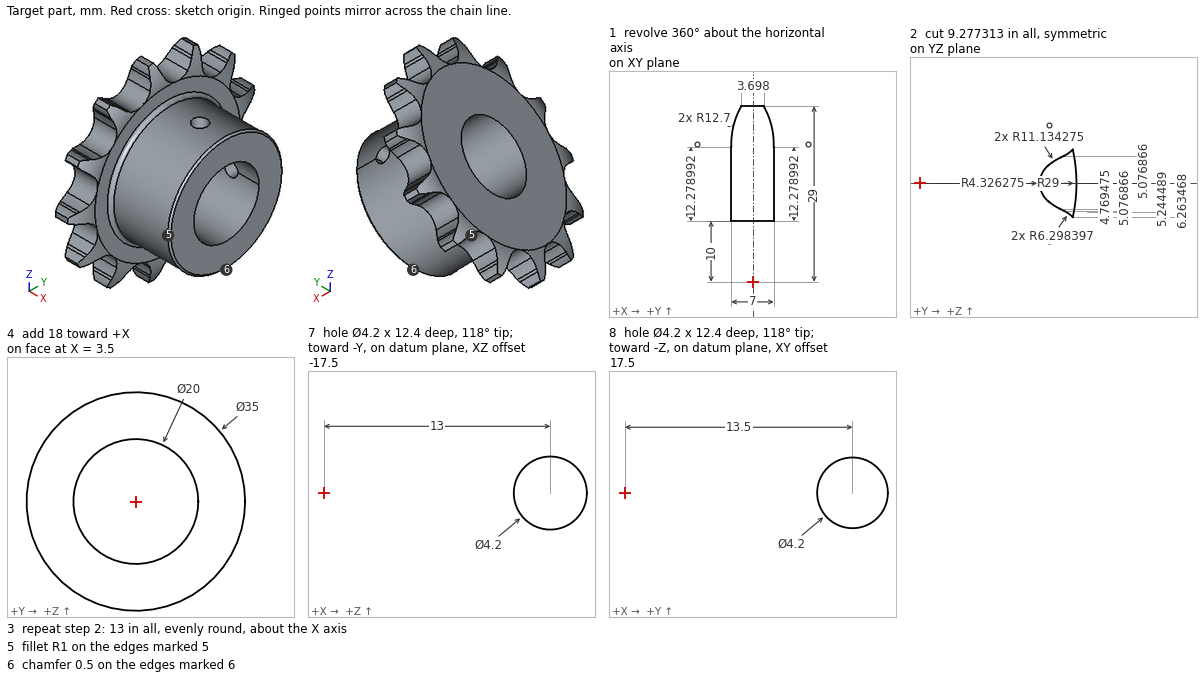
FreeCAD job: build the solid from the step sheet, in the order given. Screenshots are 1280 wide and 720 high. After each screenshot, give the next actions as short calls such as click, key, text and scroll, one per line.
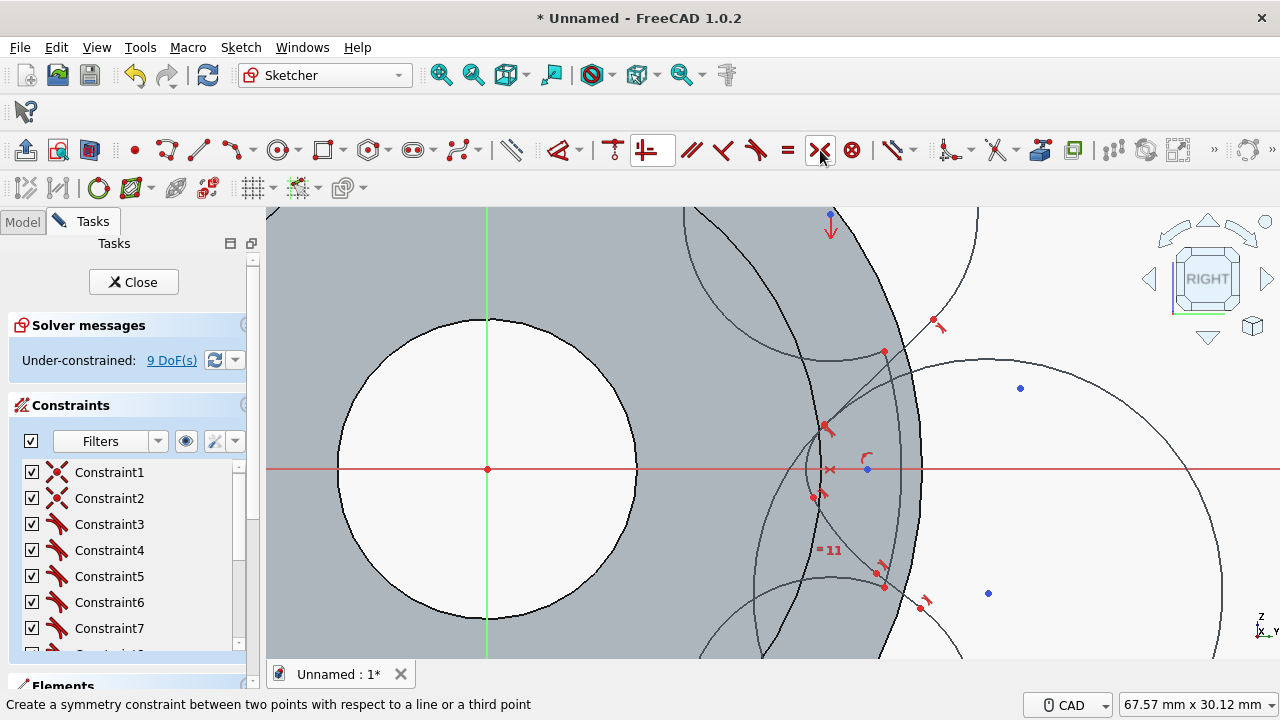
click(558, 150)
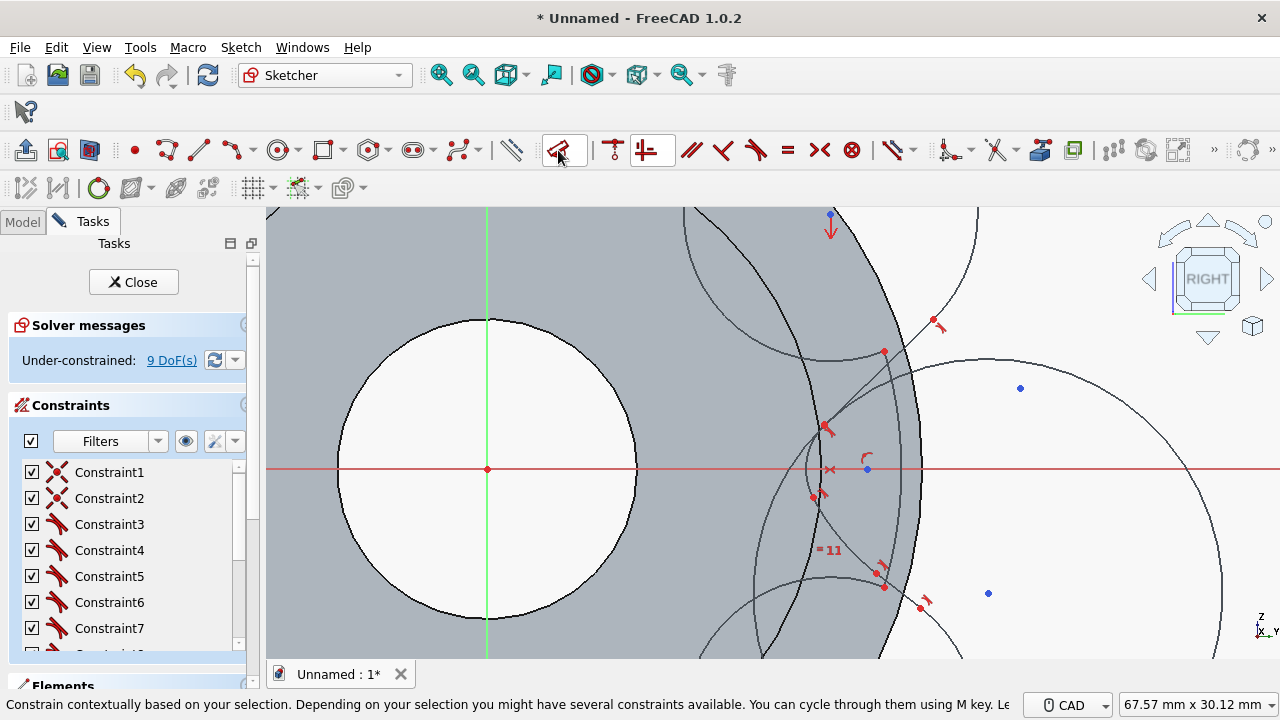
click(723, 625)
click(699, 603)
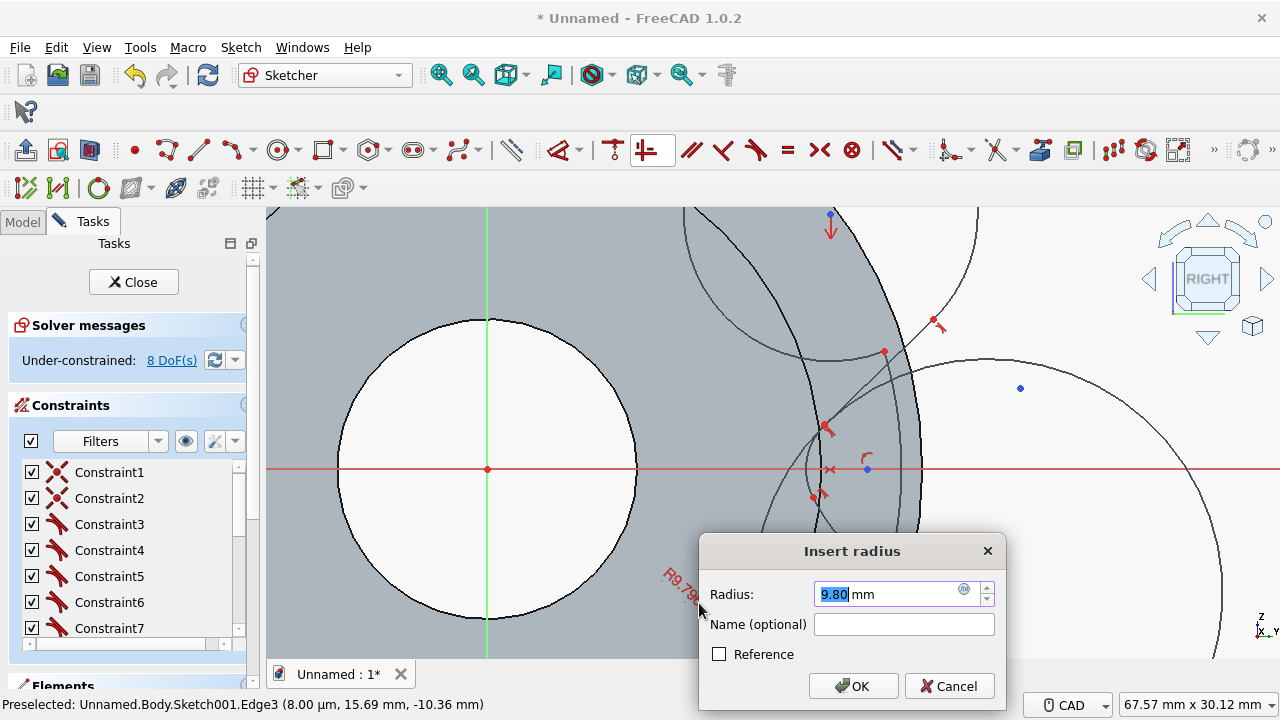
text(6.298397)
key(Return)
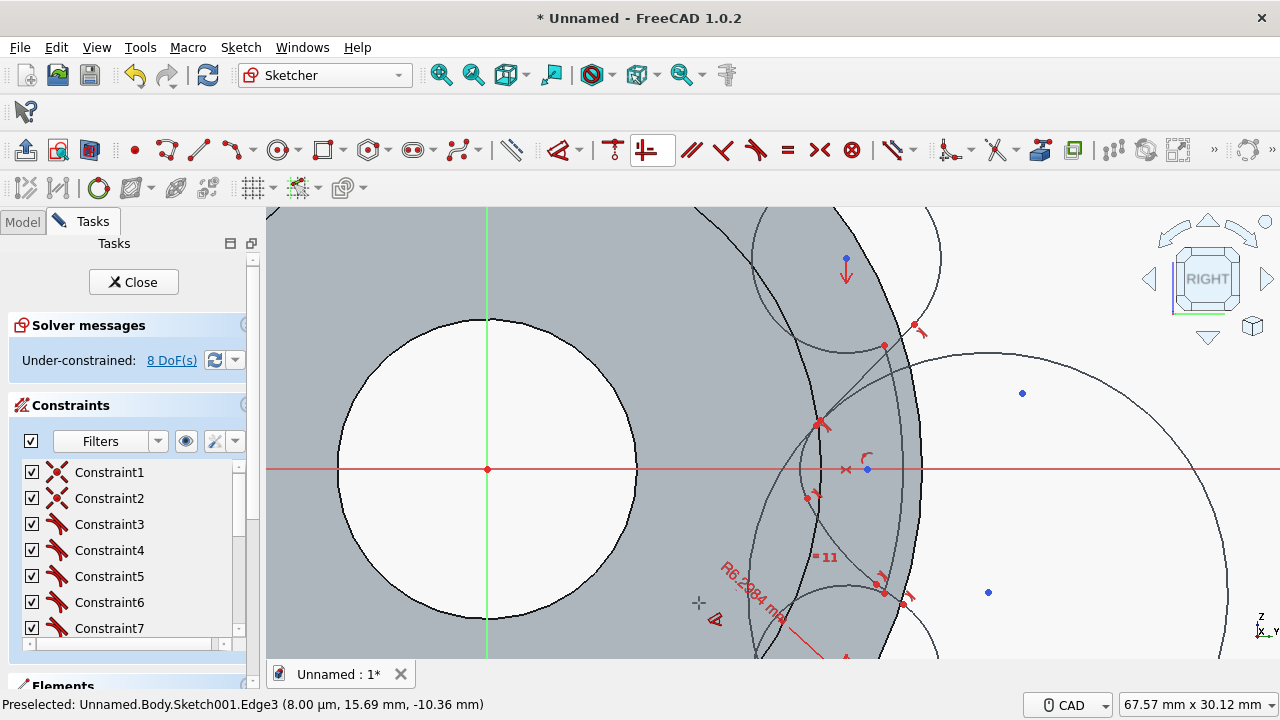
click(900, 519)
click(932, 523)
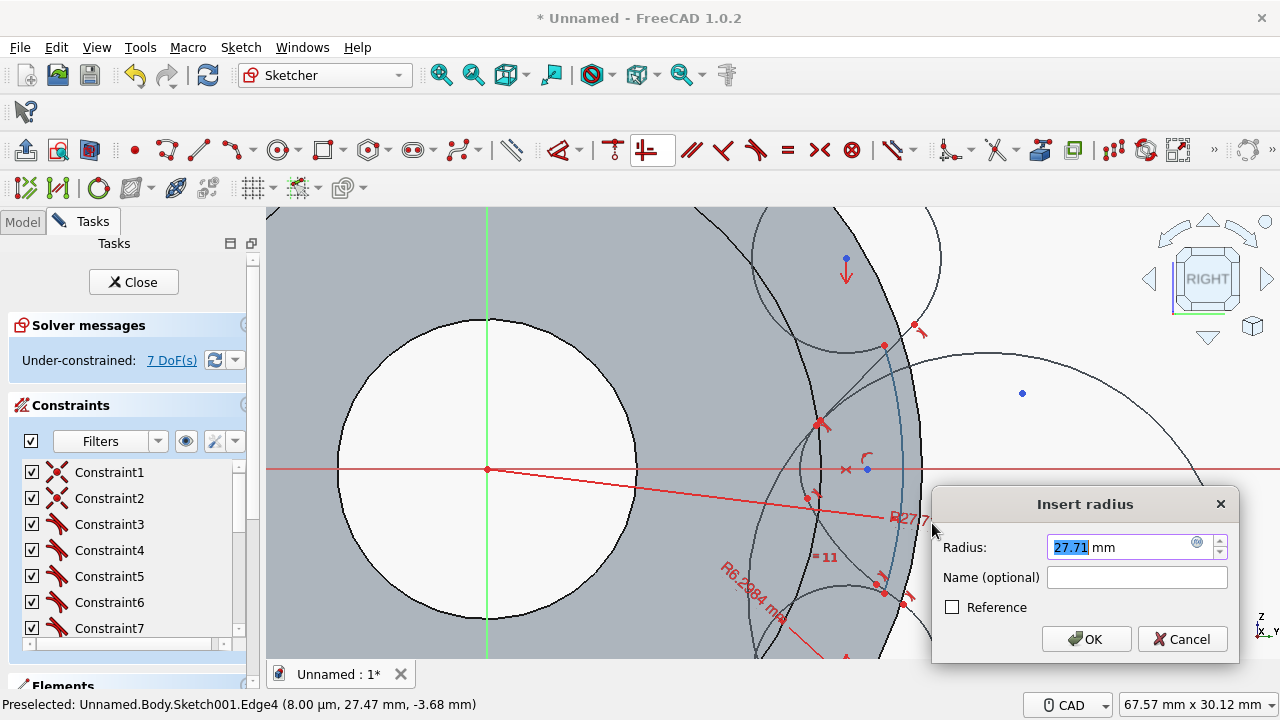
text(29)
key(Return)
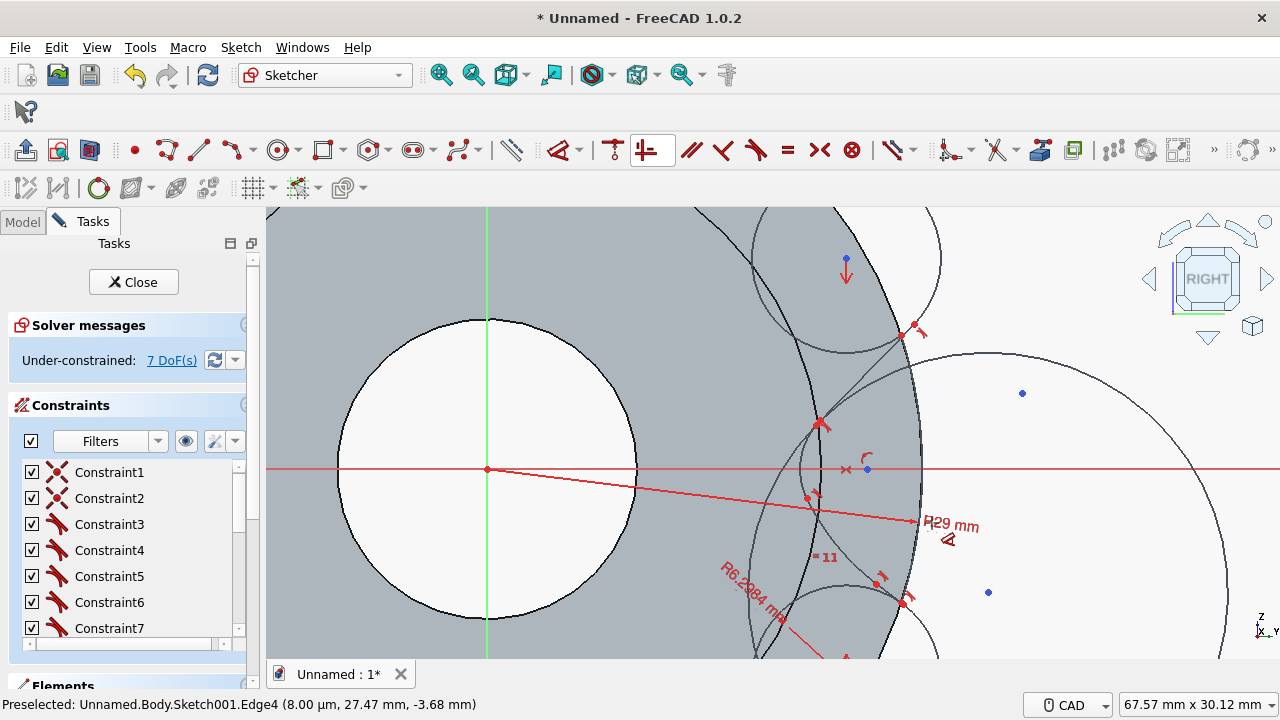
click(1099, 380)
click(1114, 352)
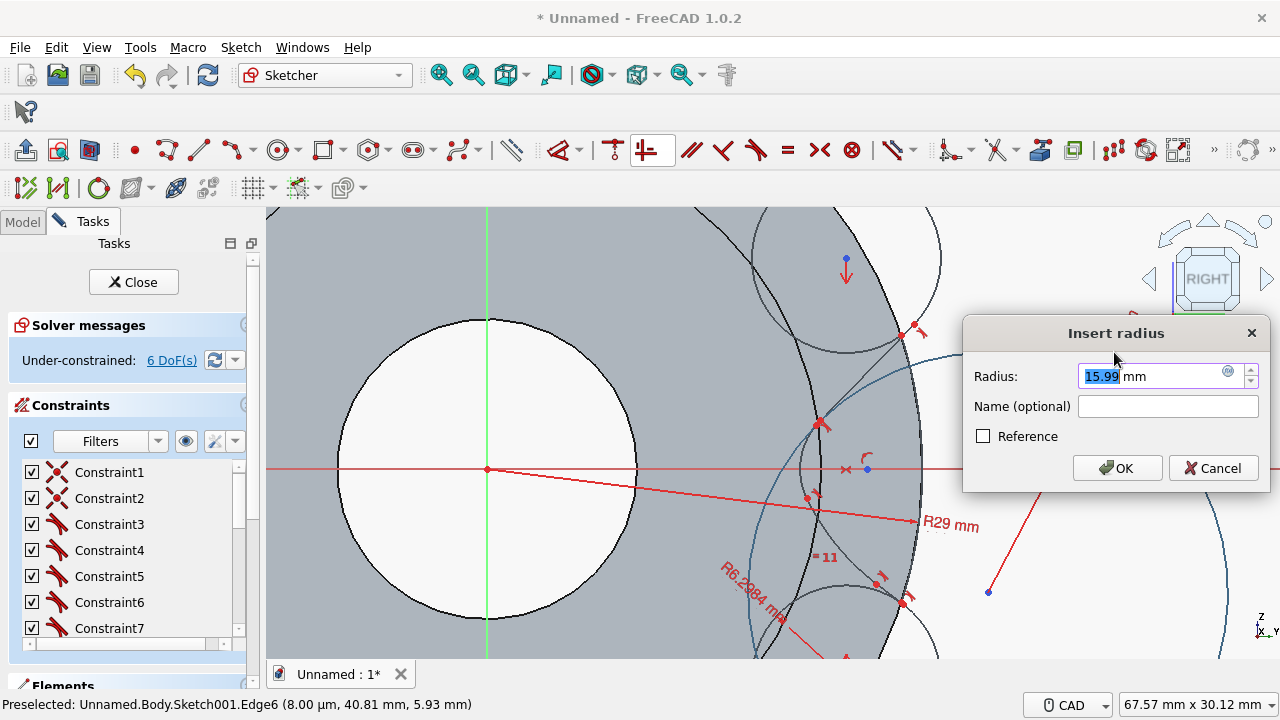
text(11.134275)
key(Return)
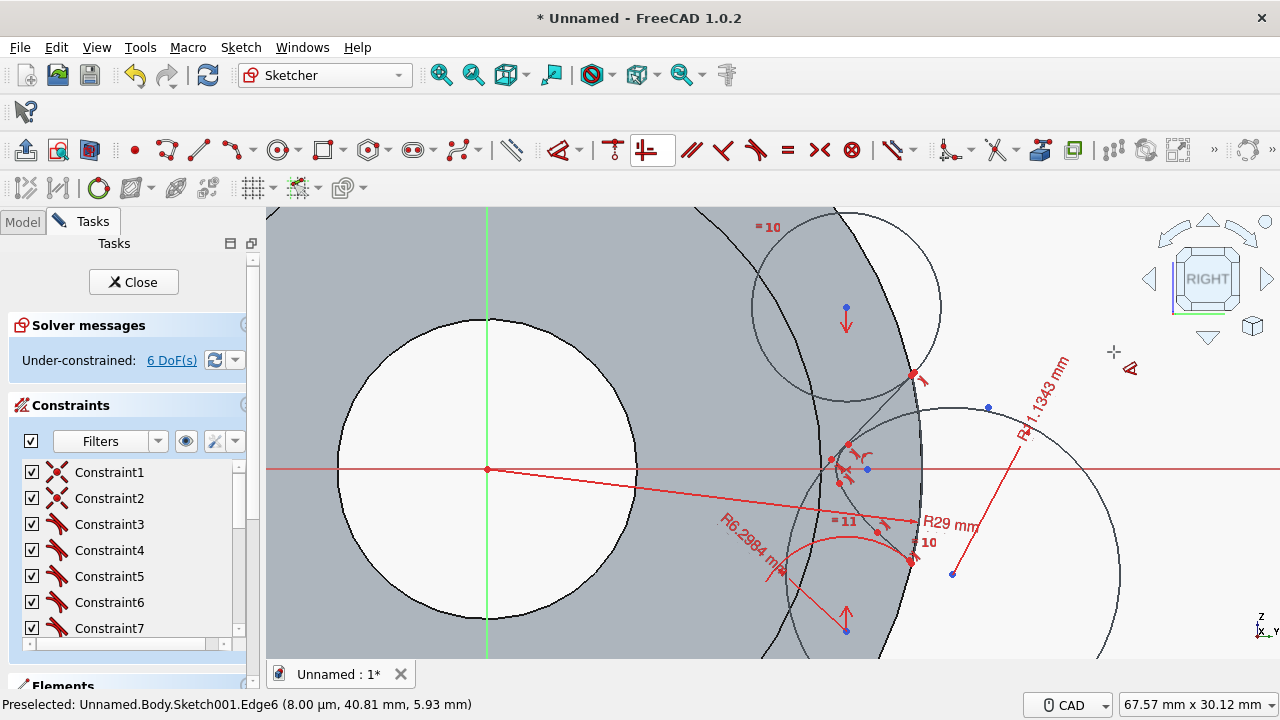
scroll(836, 471, up, 2)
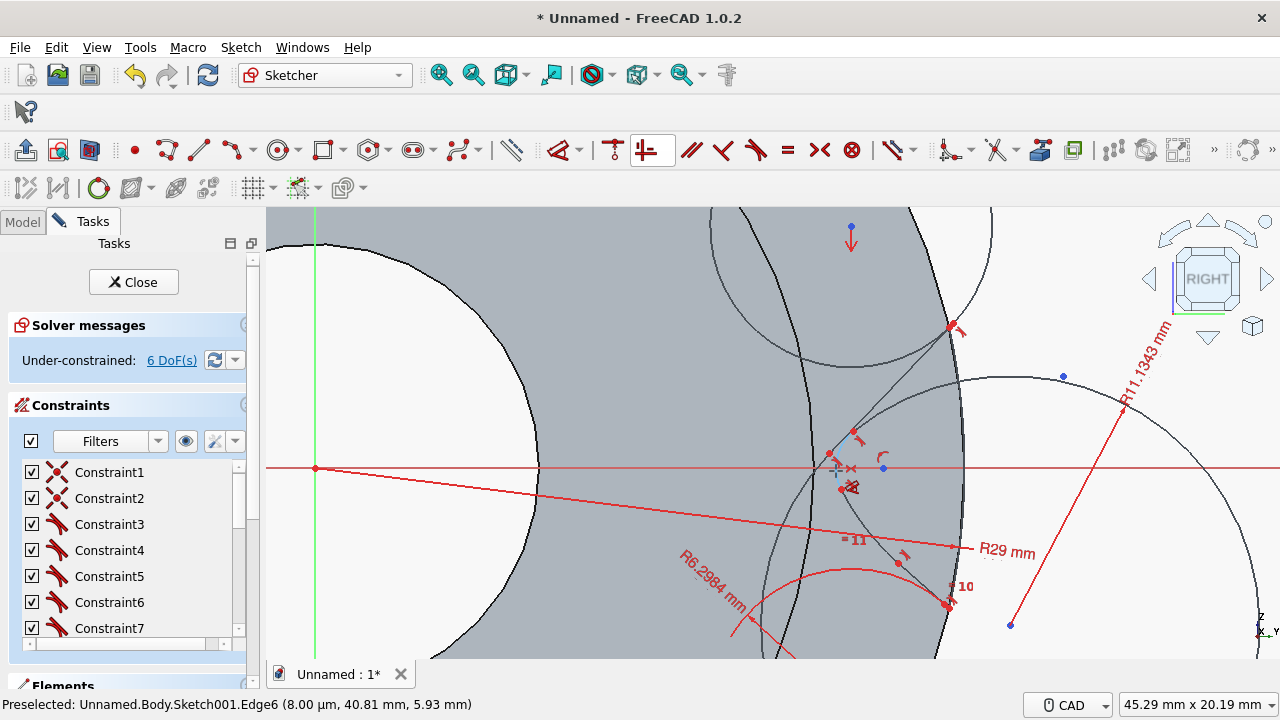
click(836, 471)
click(811, 434)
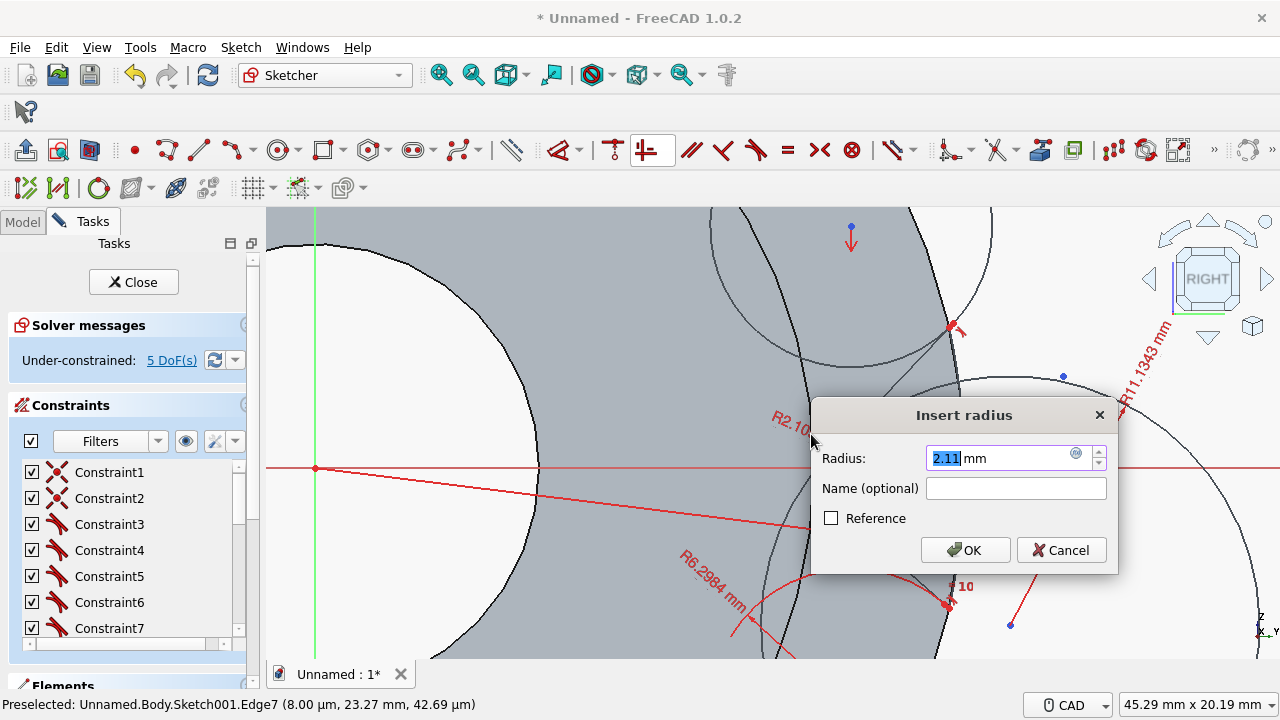
text(4.326275)
key(Return)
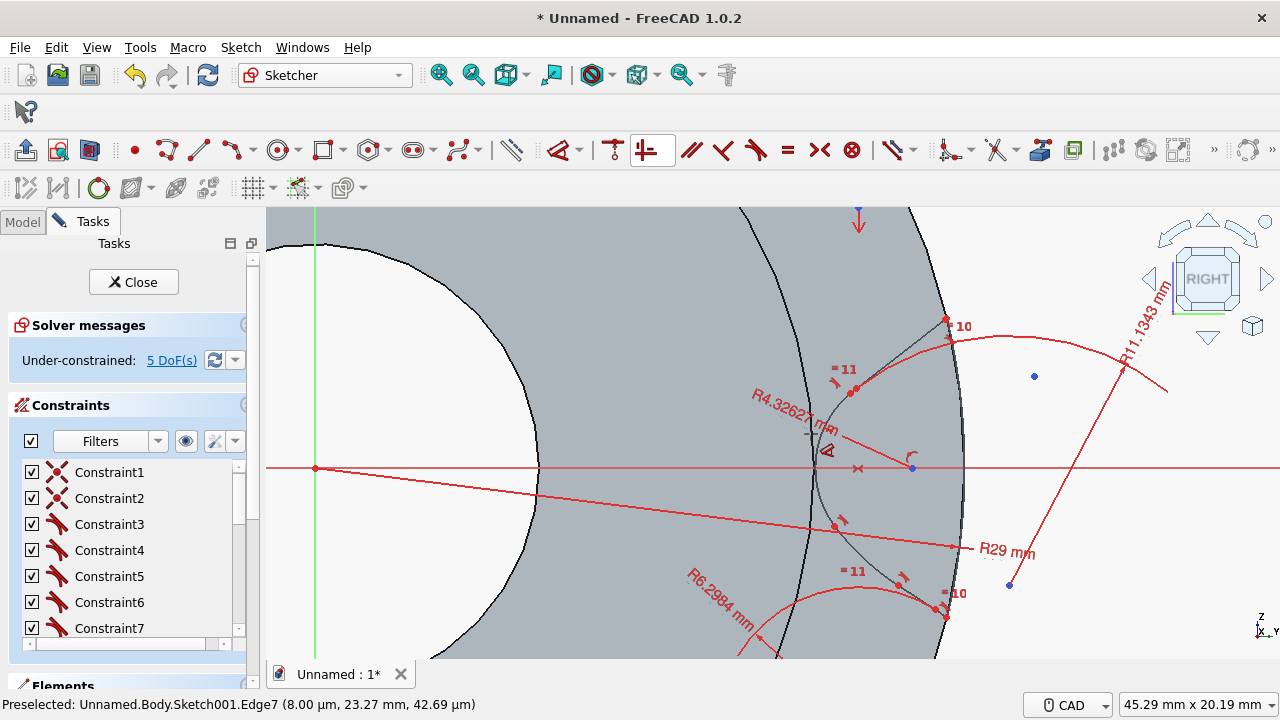
click(898, 586)
click(932, 527)